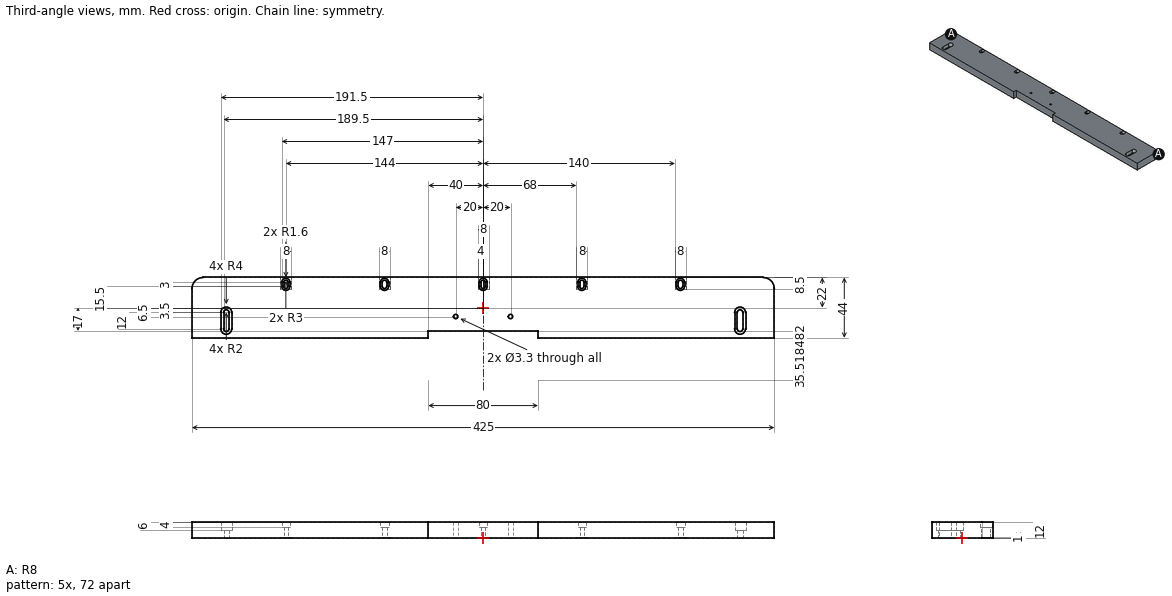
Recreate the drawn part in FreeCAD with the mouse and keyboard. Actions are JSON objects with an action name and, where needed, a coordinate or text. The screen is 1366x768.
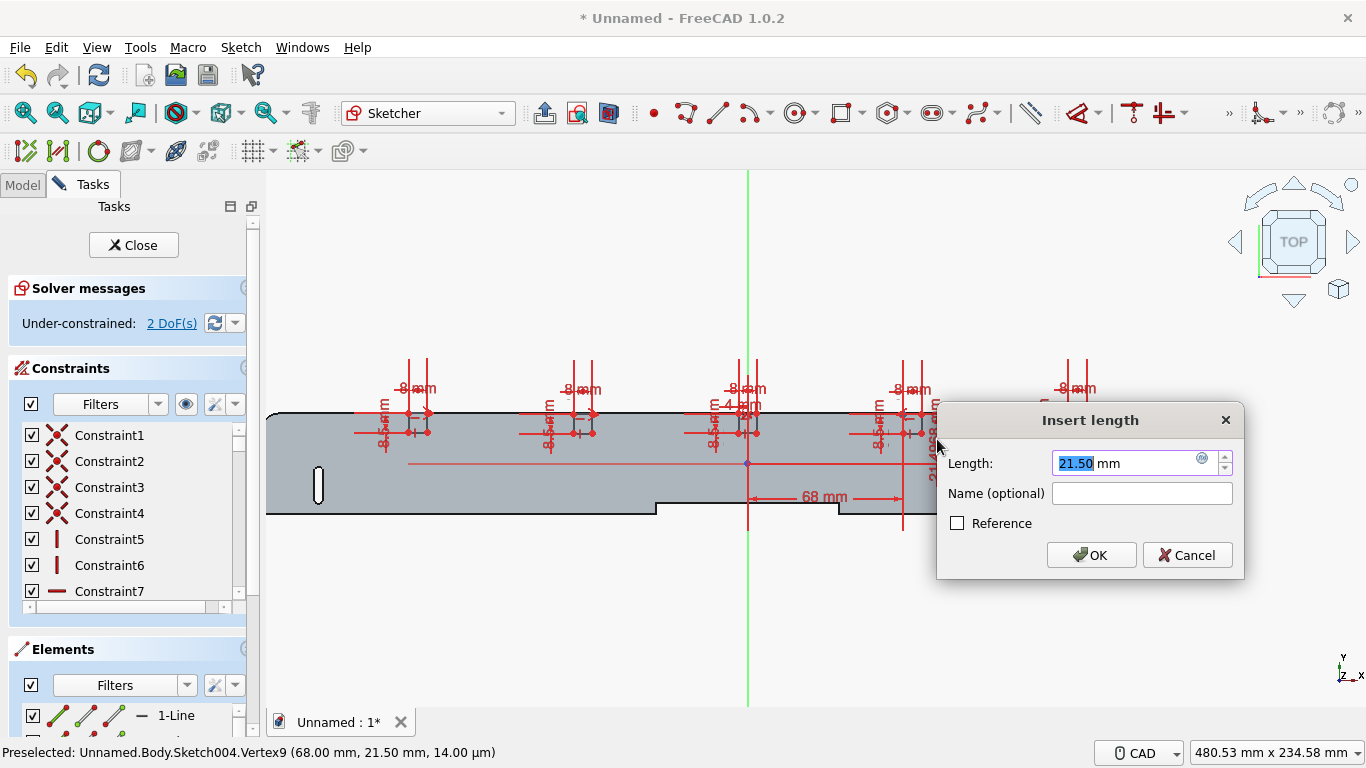
{"action": "type", "text": "22"}
{"action": "key", "text": "Return"}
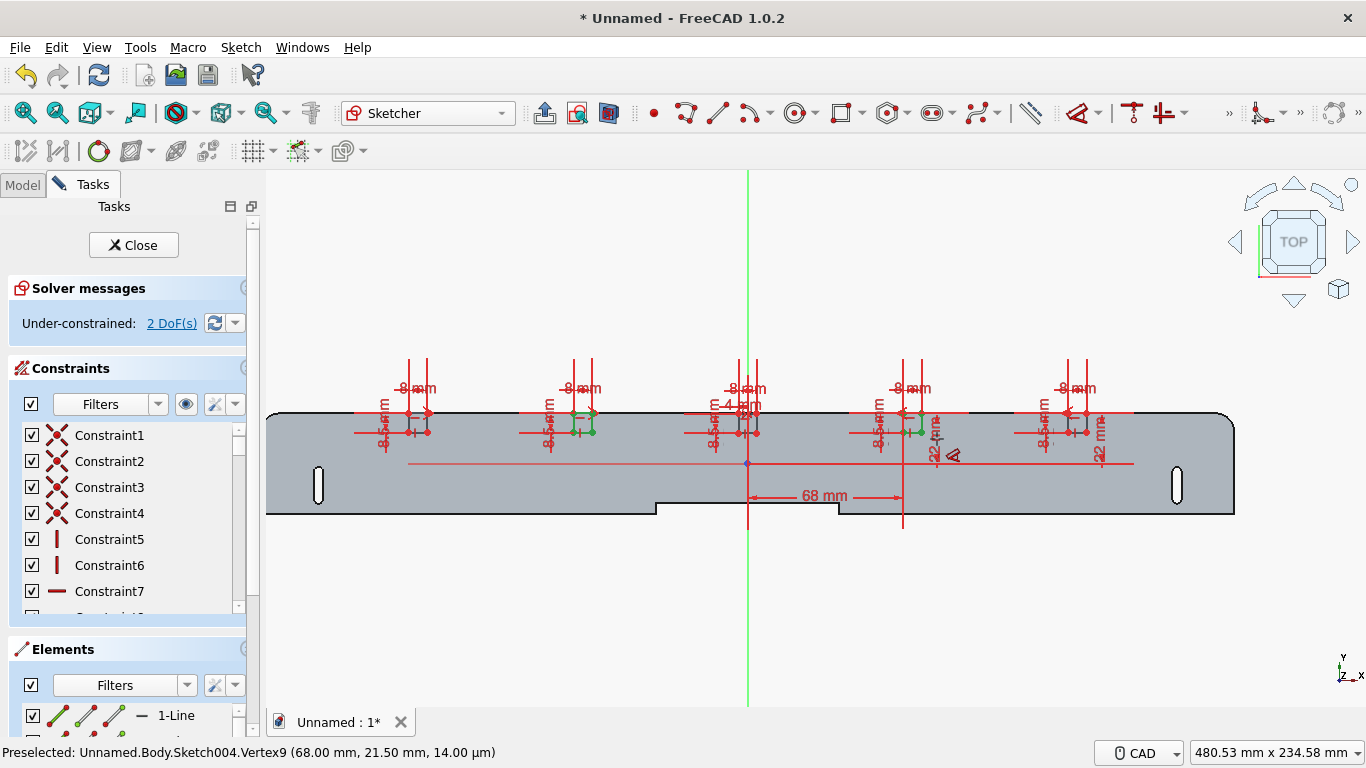
{"action": "left_click", "coordinate": [739, 414]}
{"action": "left_click", "coordinate": [705, 439]}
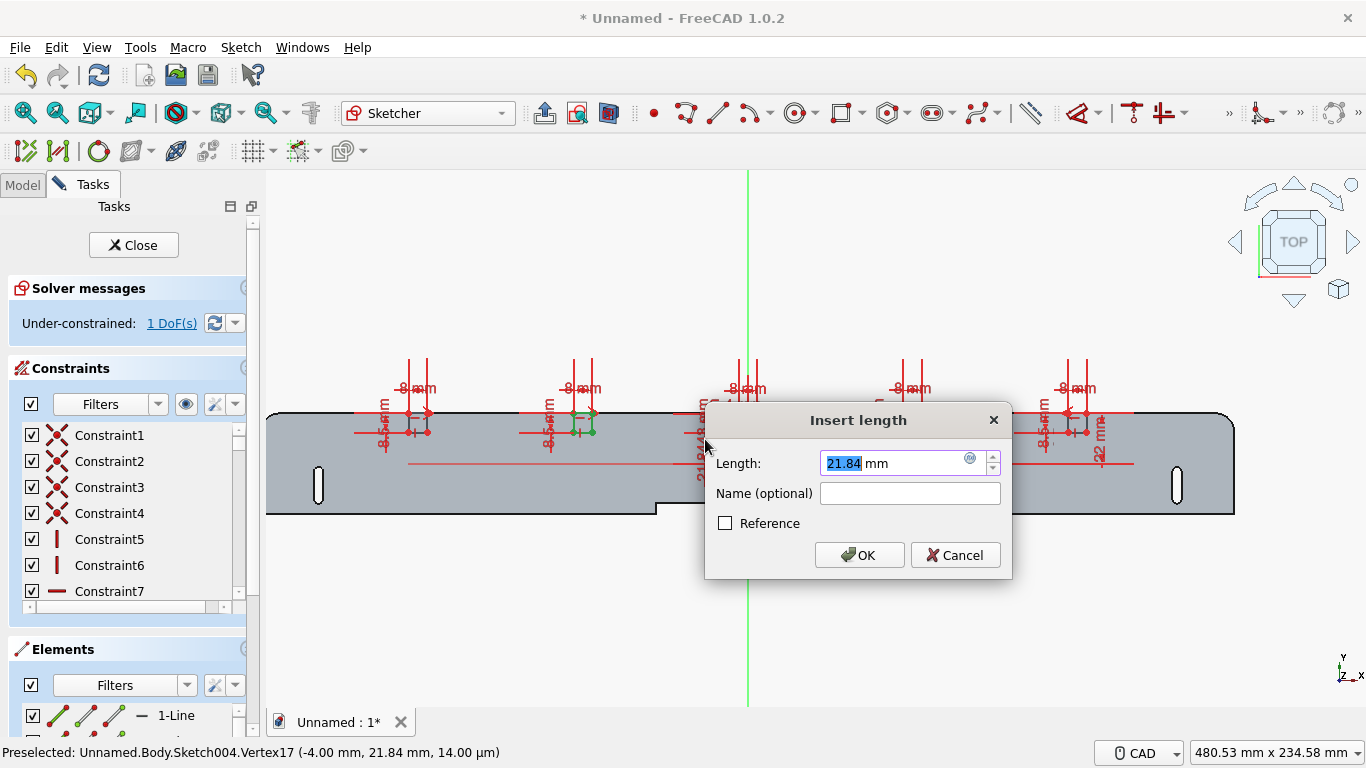
{"action": "type", "text": "22"}
{"action": "key", "text": "Return"}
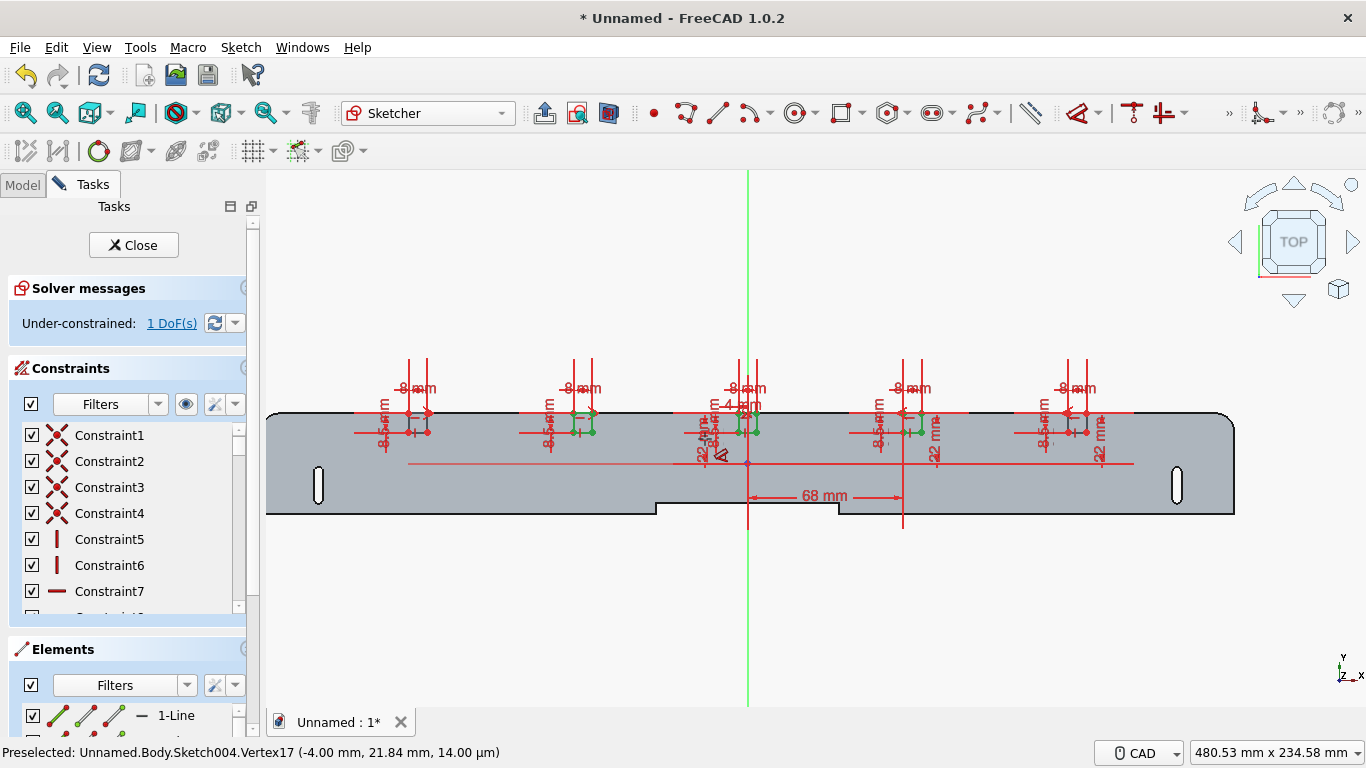
{"action": "left_click", "coordinate": [1068, 413]}
{"action": "left_click", "coordinate": [908, 498]}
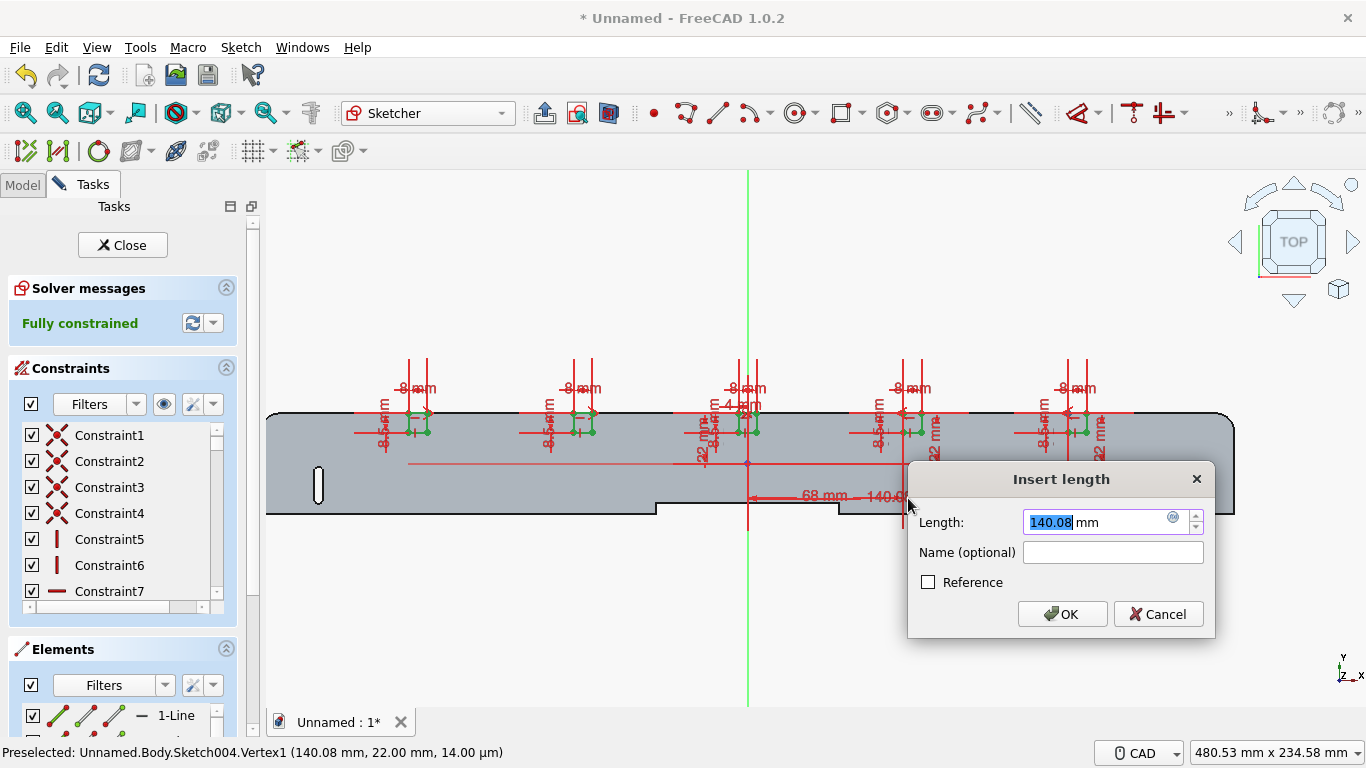
{"action": "type", "text": "140"}
{"action": "key", "text": "Return"}
{"action": "key", "text": "Escape"}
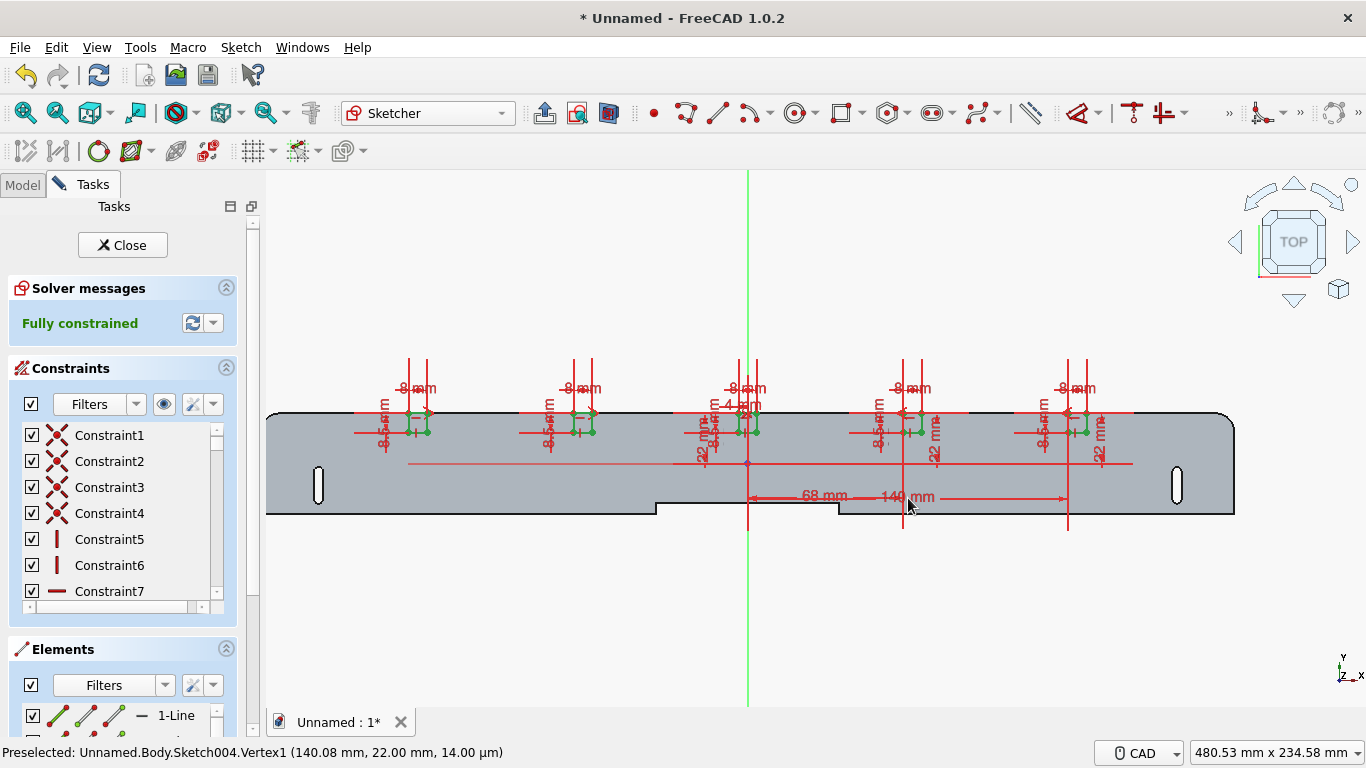
{"action": "left_click", "coordinate": [123, 245]}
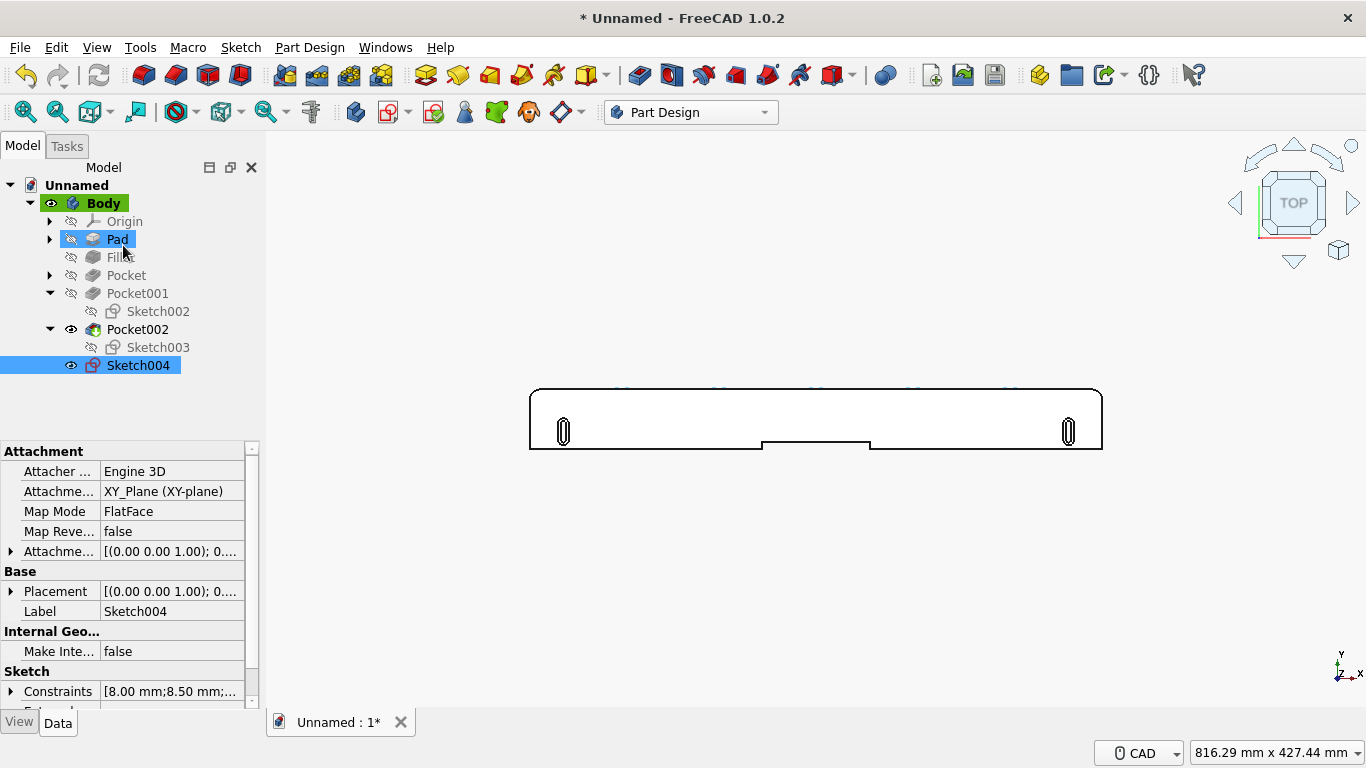
{"action": "left_click", "coordinate": [640, 76]}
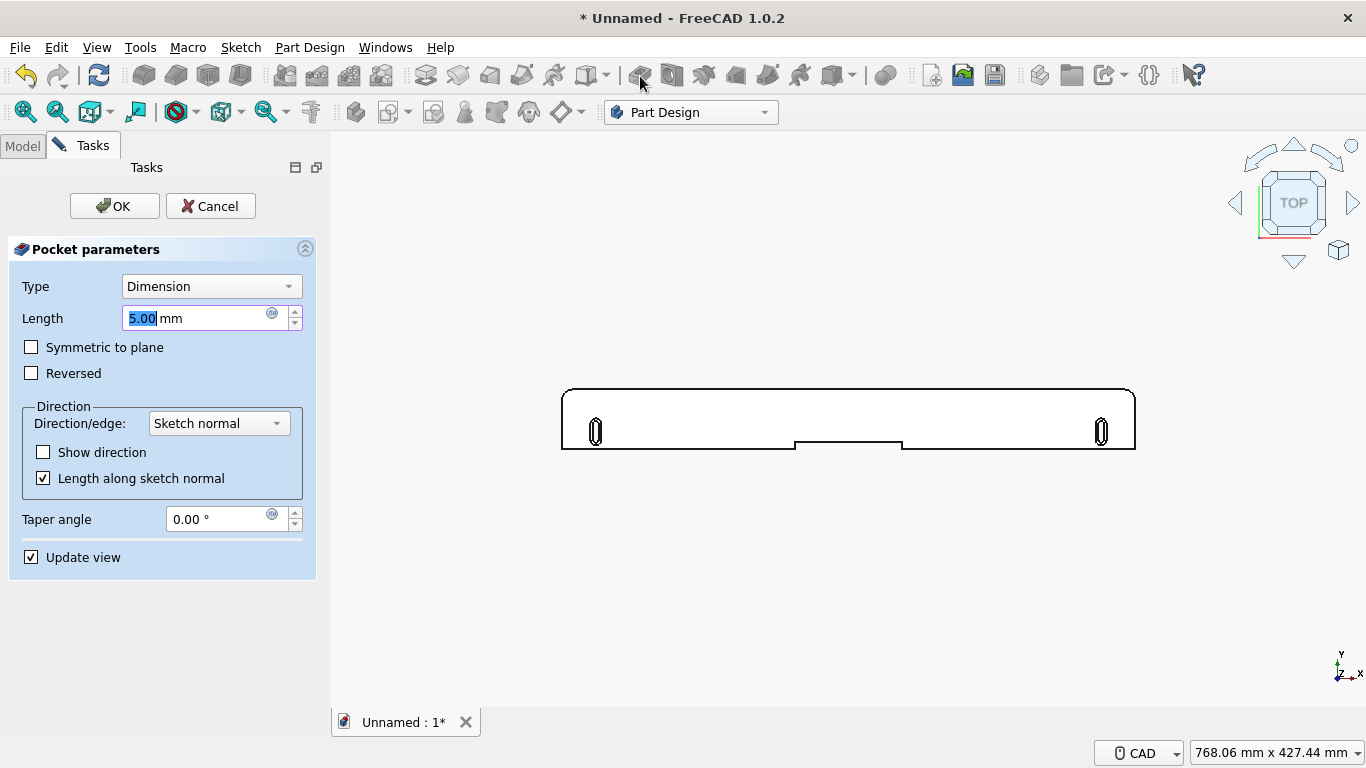
{"action": "type", "text": "1"}
{"action": "key", "text": "Tab"}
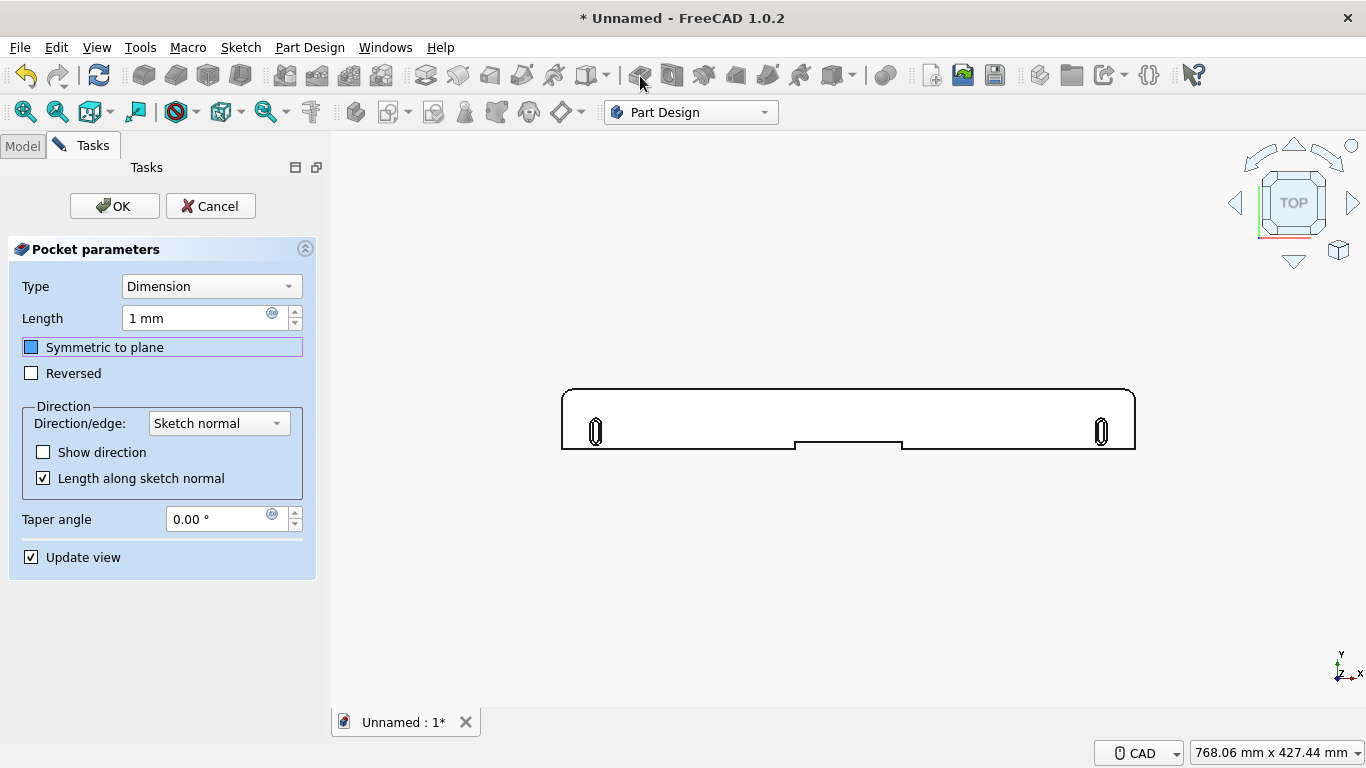
{"action": "left_click", "coordinate": [30, 373]}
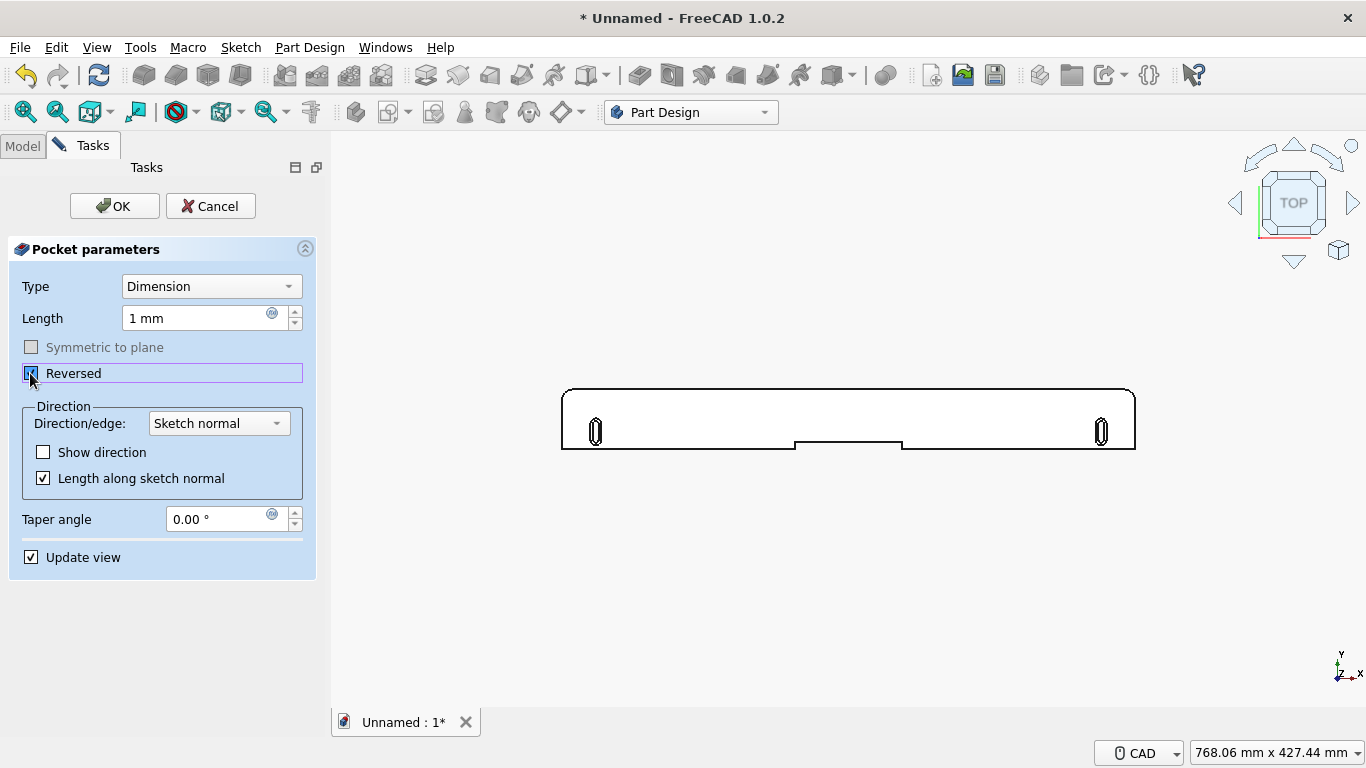
{"action": "left_click", "coordinate": [115, 206]}